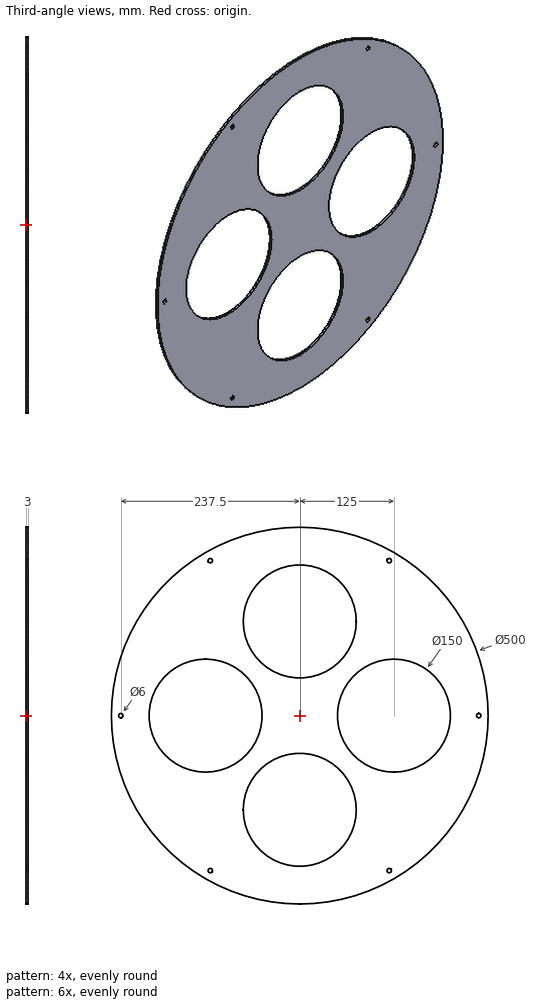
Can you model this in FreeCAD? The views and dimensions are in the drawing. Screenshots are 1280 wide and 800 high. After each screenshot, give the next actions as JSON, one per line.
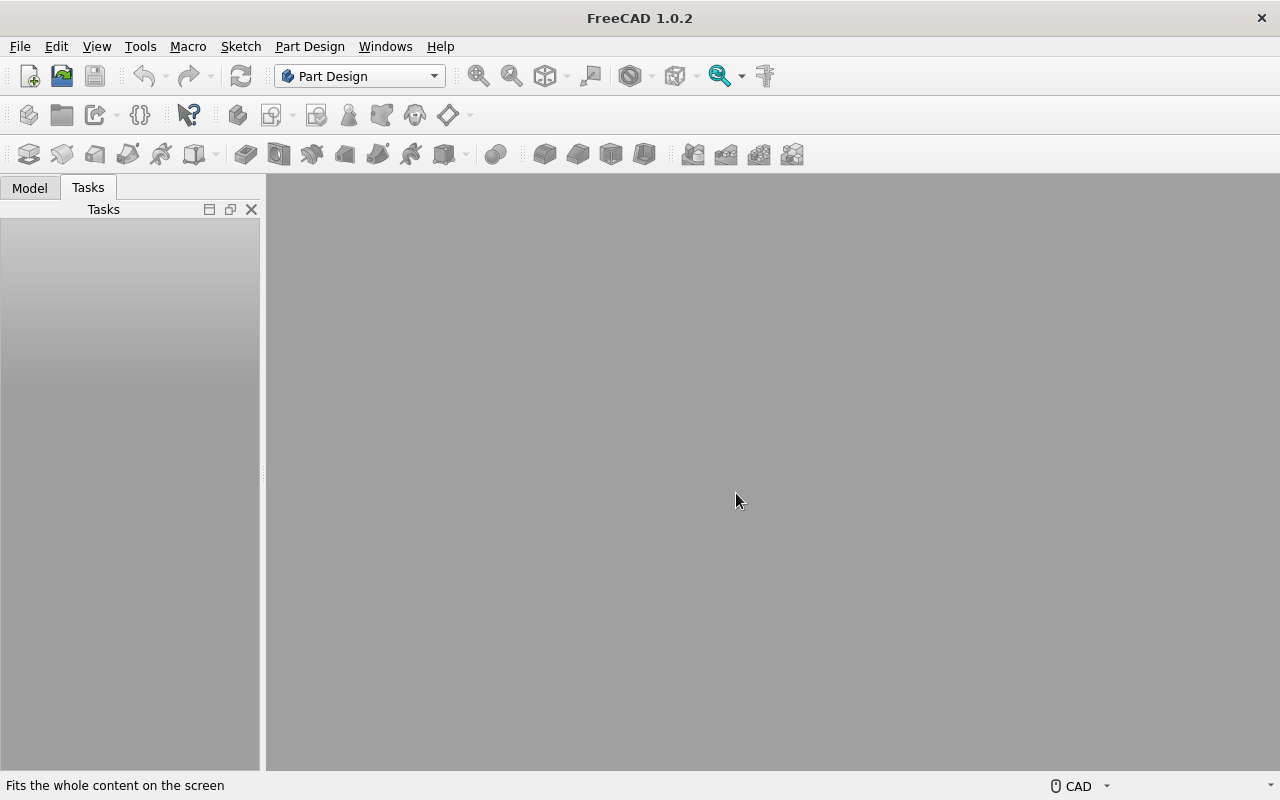
{"action": "left_click", "coordinate": [29, 76]}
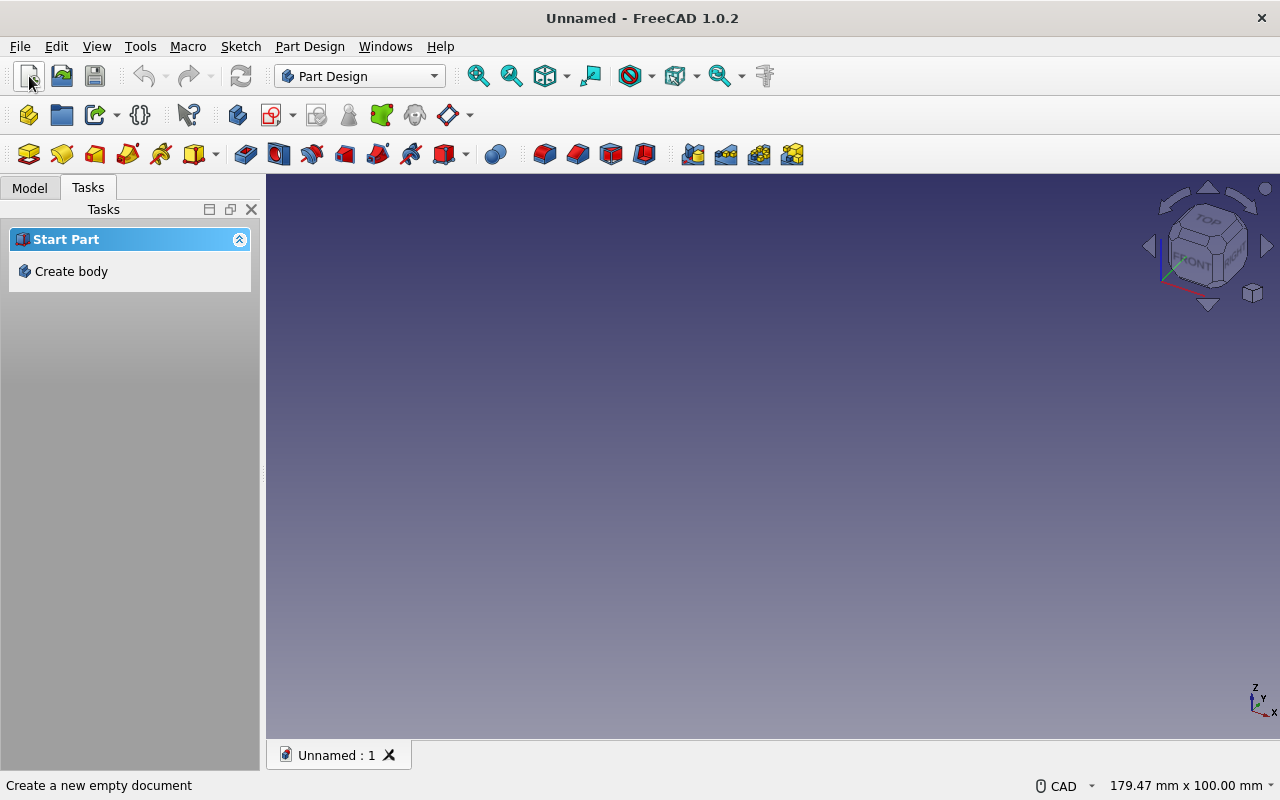
{"action": "left_click", "coordinate": [270, 116]}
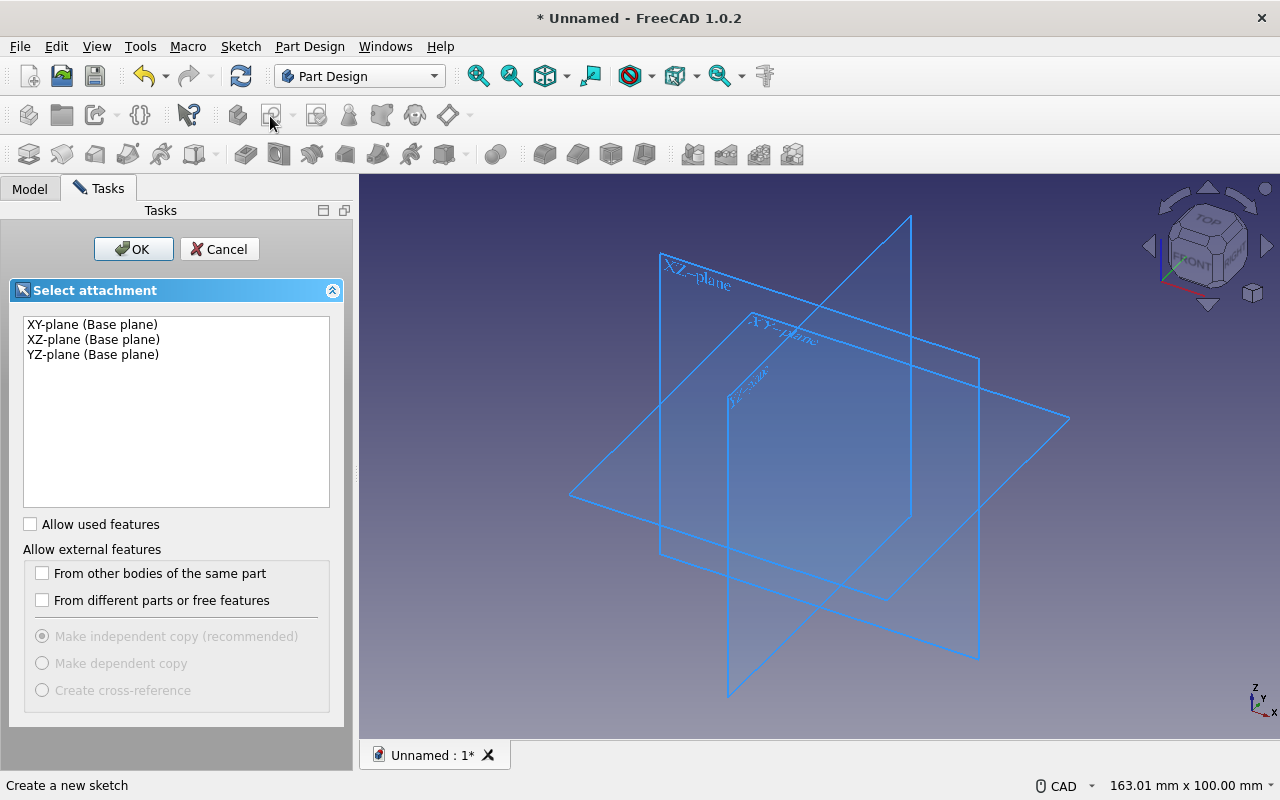
{"action": "left_click", "coordinate": [84, 354]}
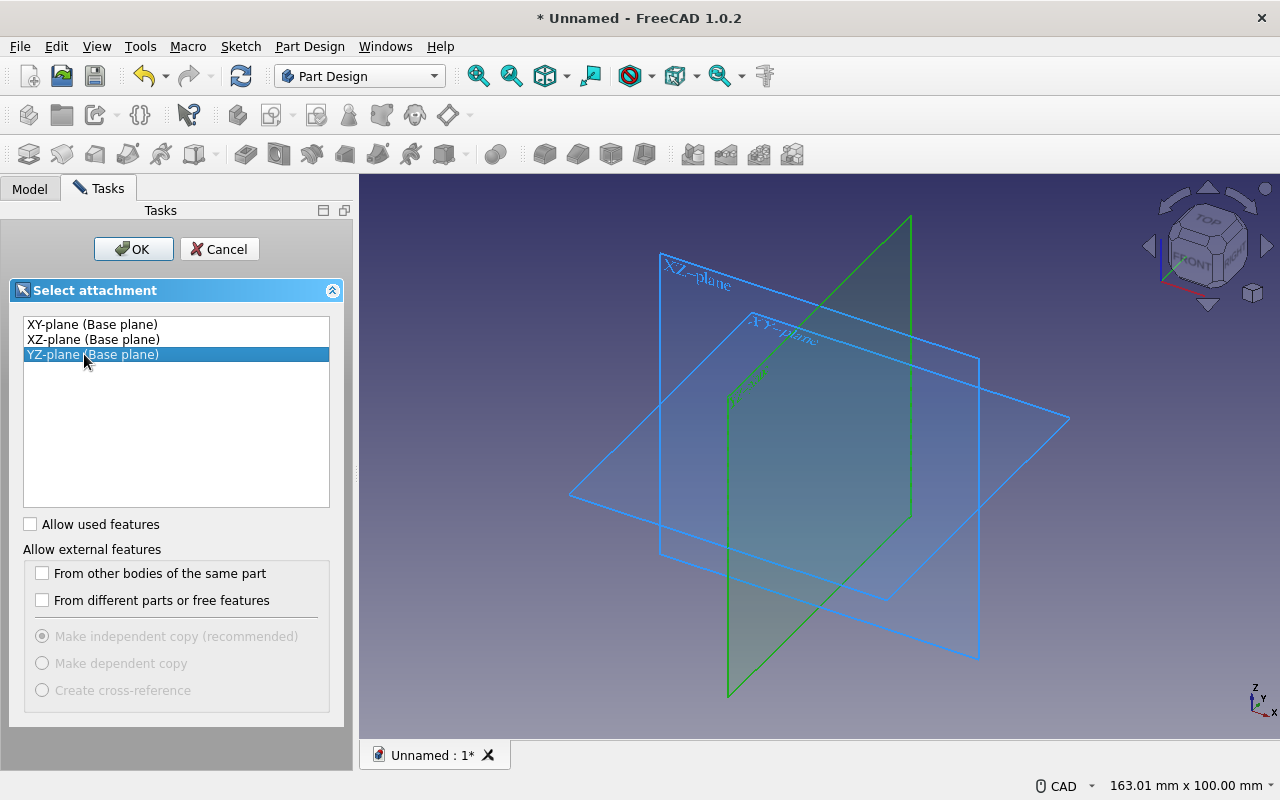
{"action": "left_click", "coordinate": [134, 249]}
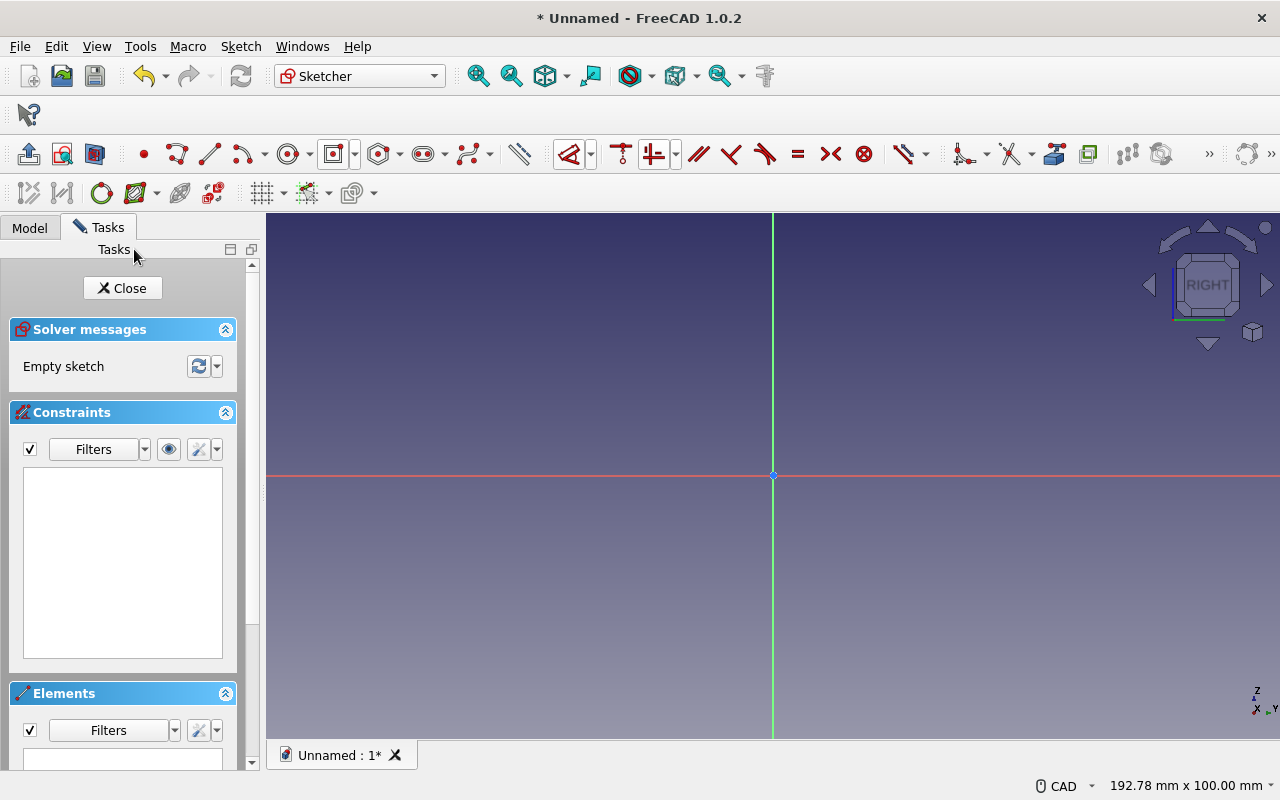
{"action": "scroll", "coordinate": [694, 476], "scroll_direction": "down", "scroll_amount": 10}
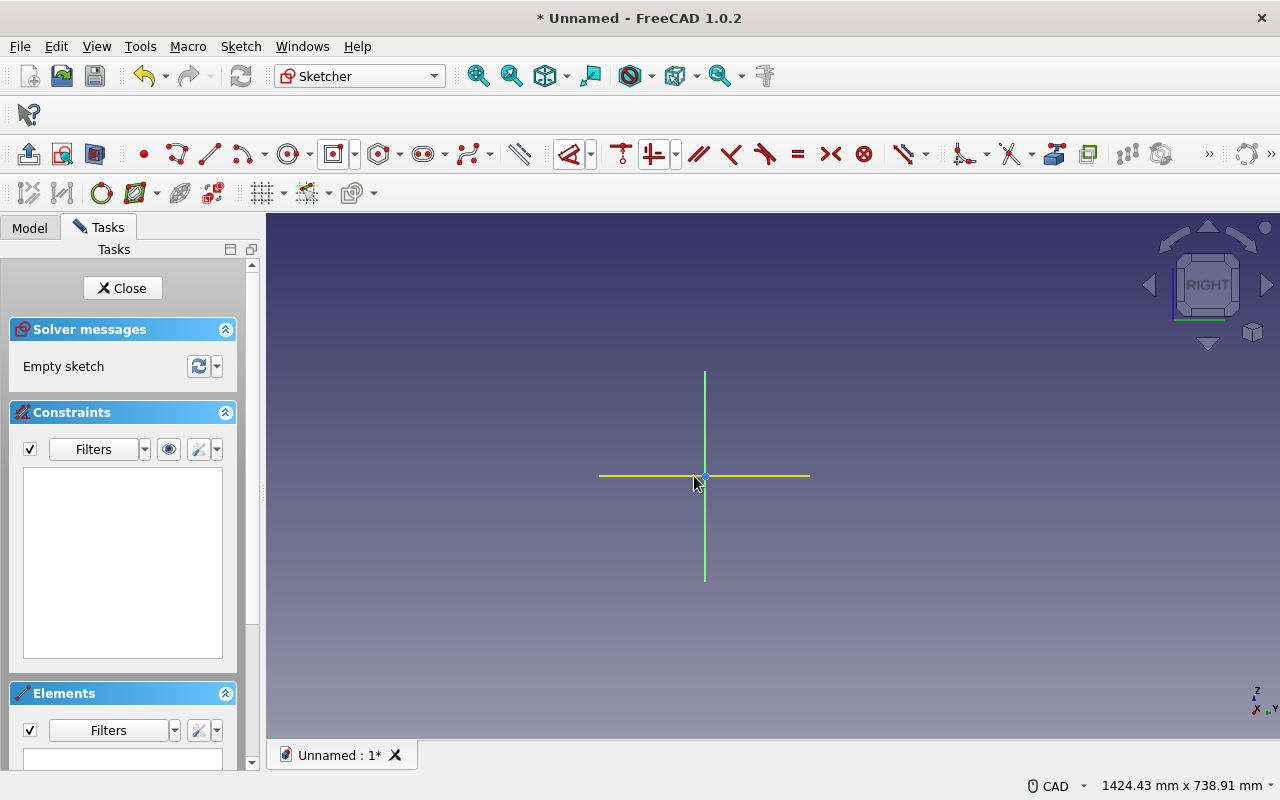
{"action": "left_click", "coordinate": [288, 154]}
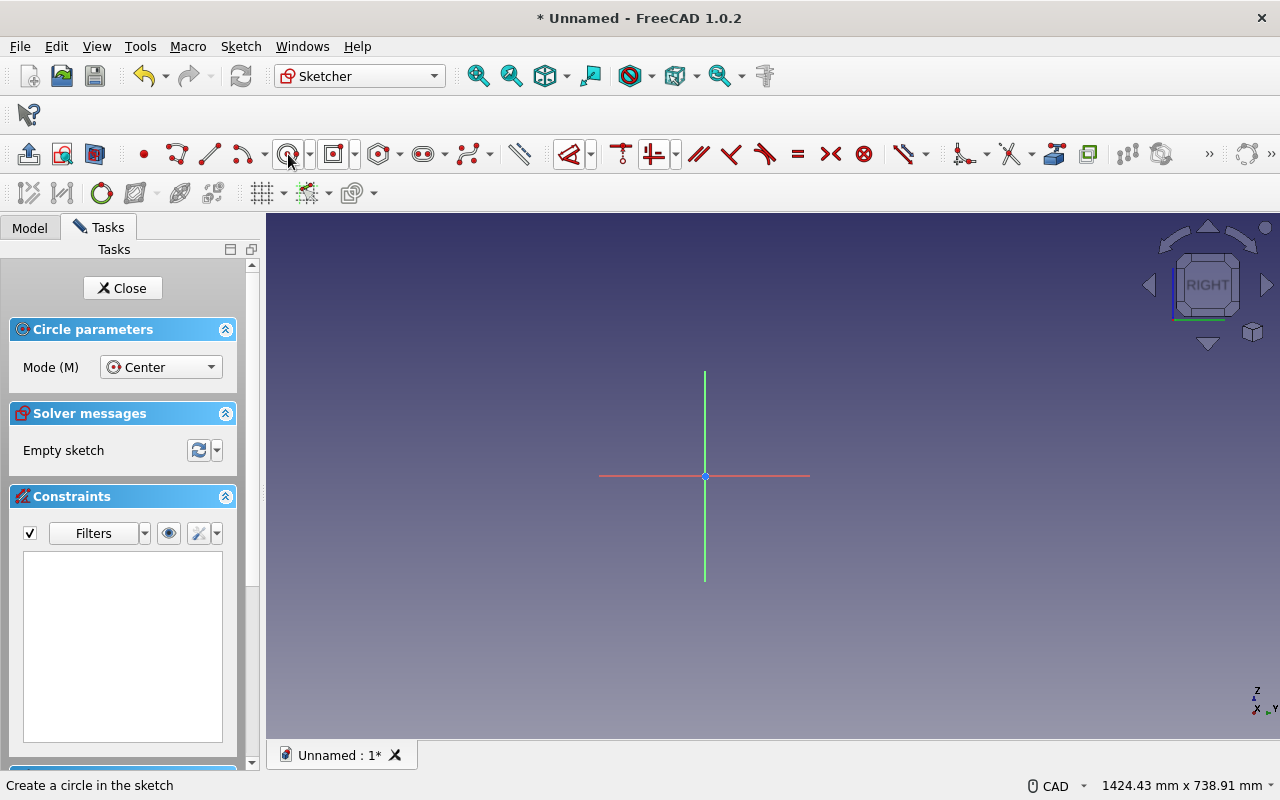
{"action": "left_click", "coordinate": [705, 476]}
{"action": "mouse_move", "coordinate": [831, 351]}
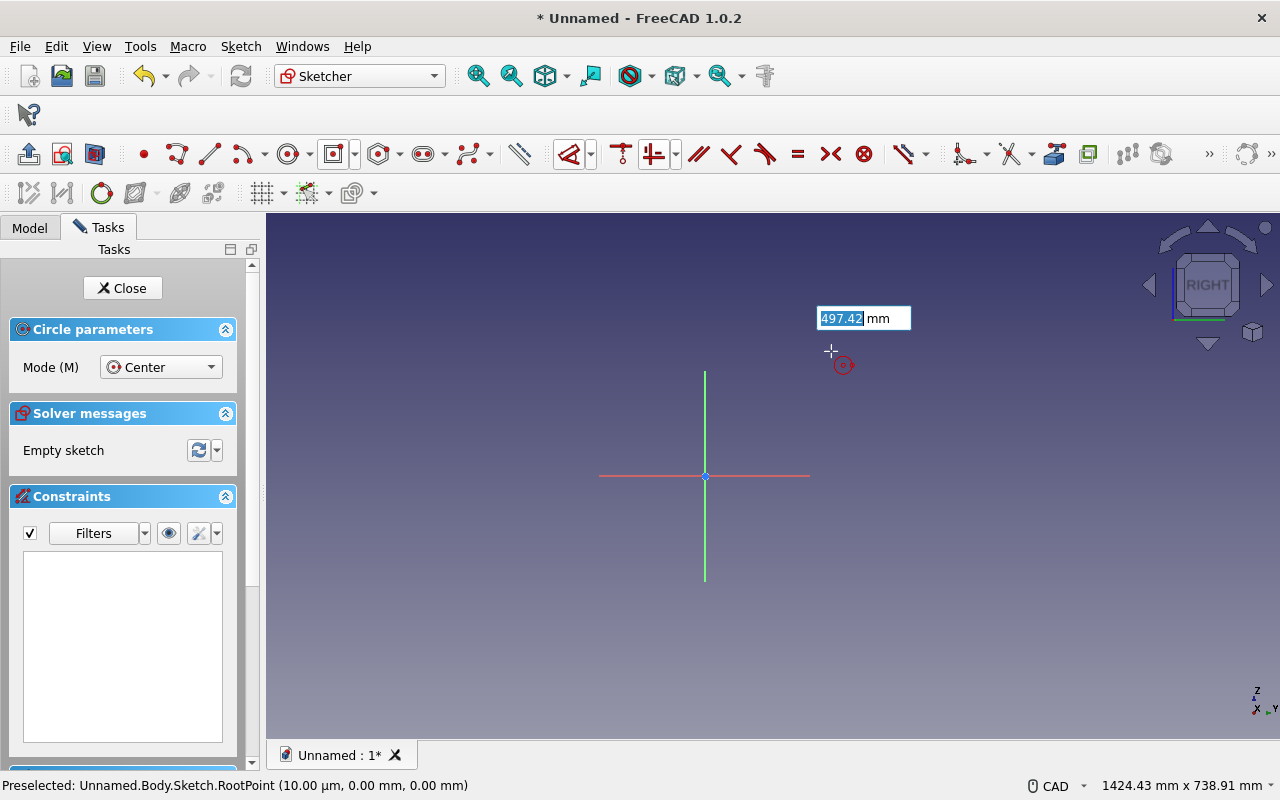
{"action": "type", "text": "500"}
{"action": "key", "text": "Return"}
{"action": "key", "text": "Escape"}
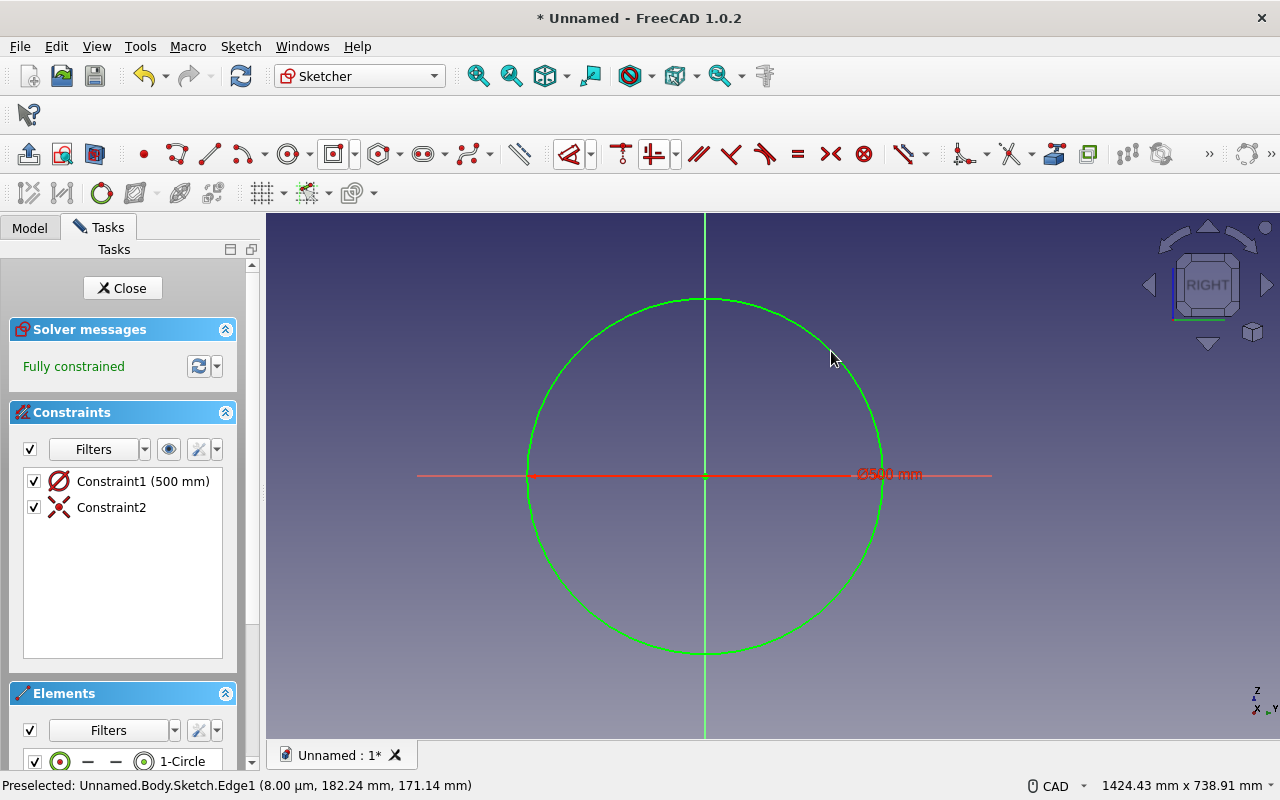
{"action": "left_click", "coordinate": [123, 288]}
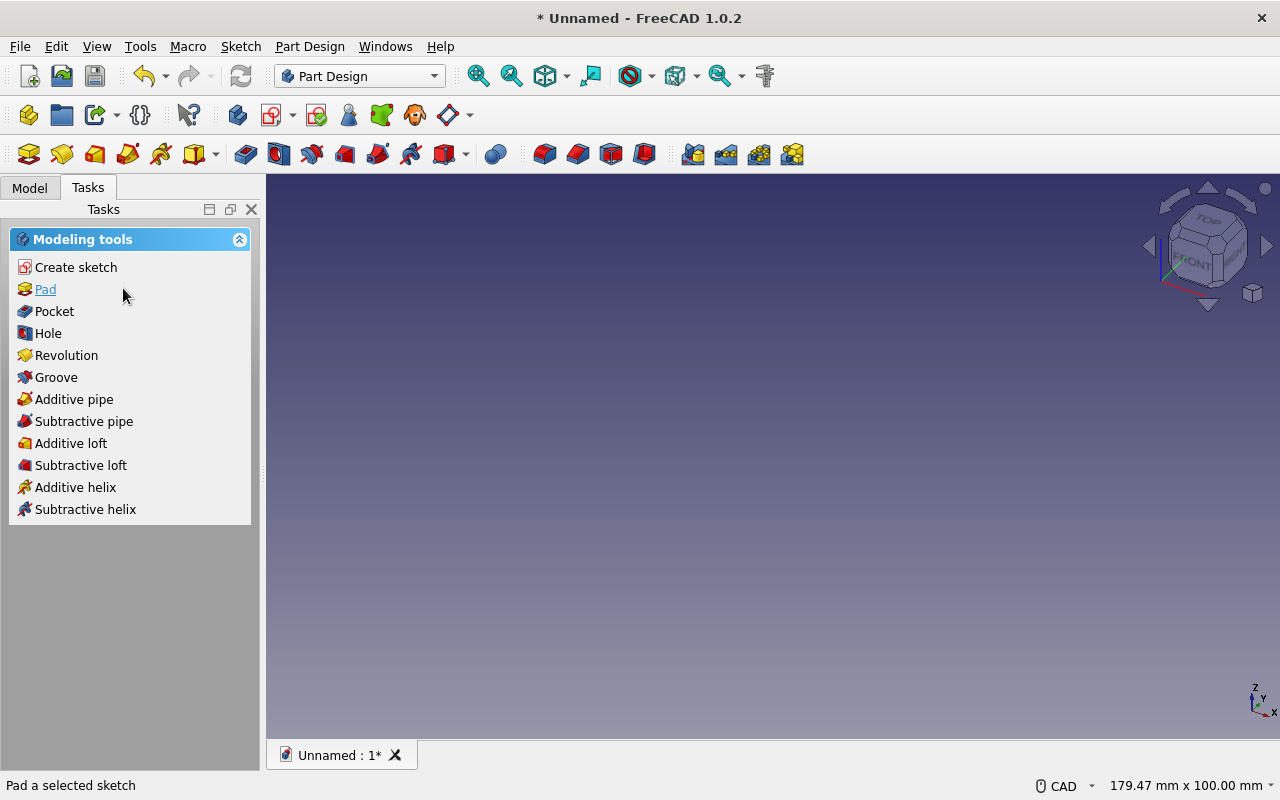
{"action": "left_click", "coordinate": [29, 154]}